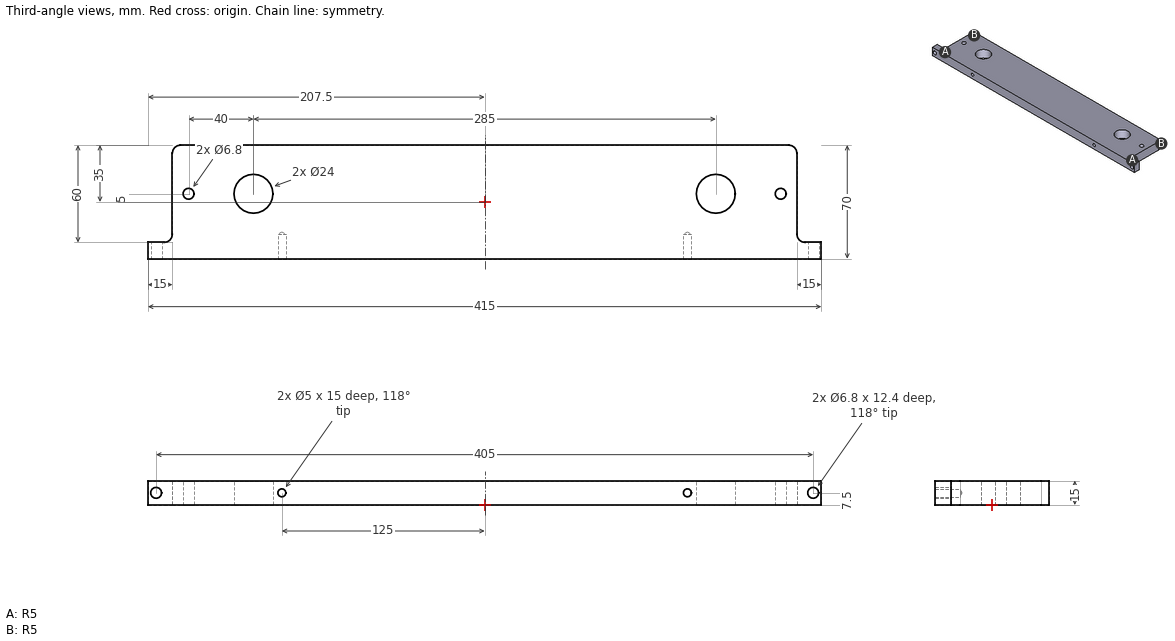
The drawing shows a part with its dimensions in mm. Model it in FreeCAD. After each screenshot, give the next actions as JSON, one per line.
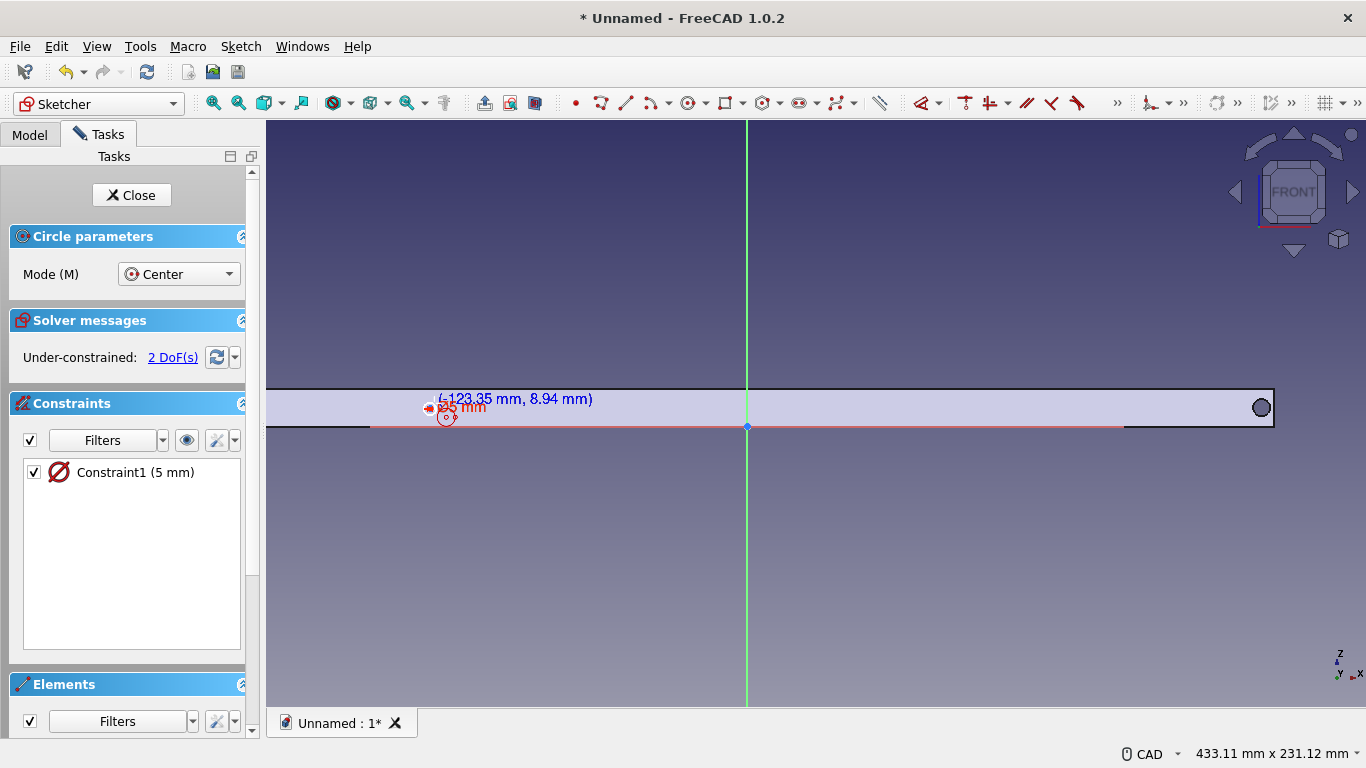
{"action": "scroll", "coordinate": [1065, 408], "scroll_direction": "up", "scroll_amount": 7}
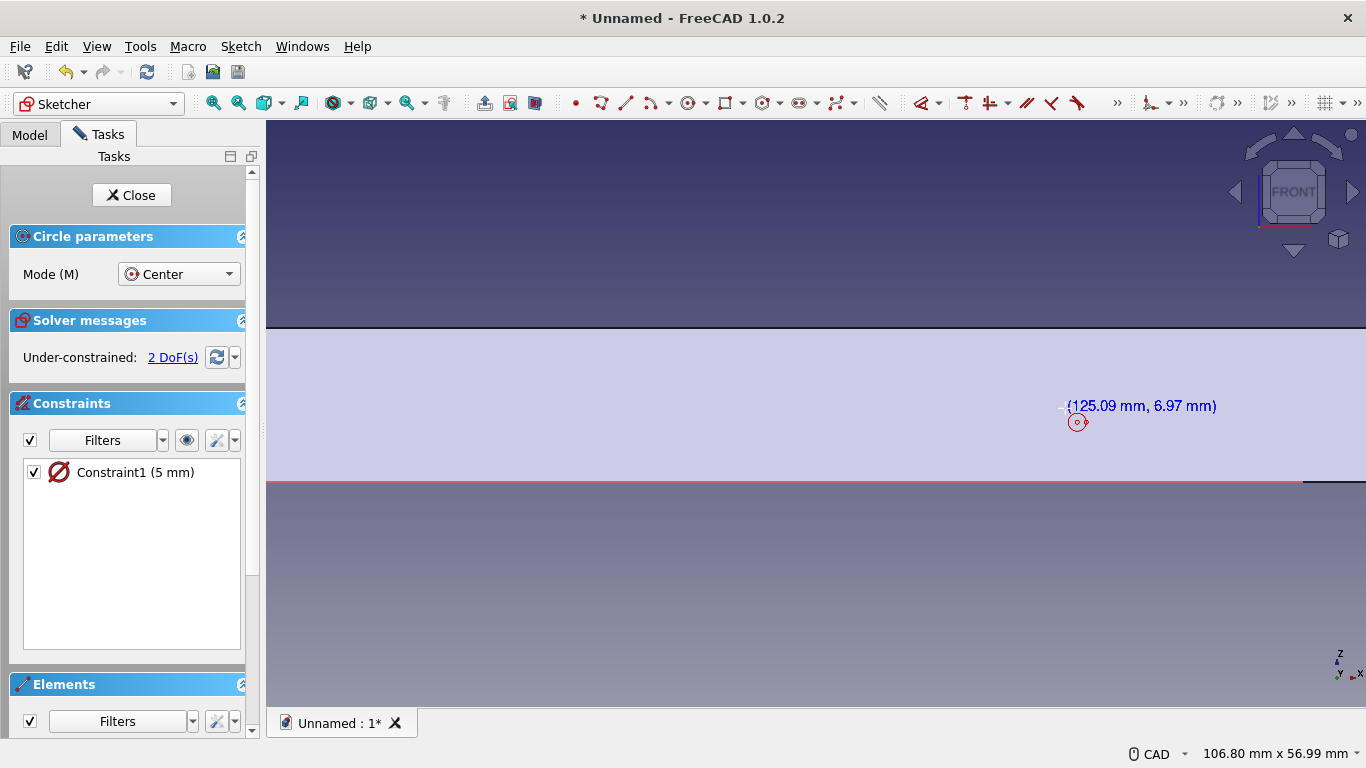
{"action": "scroll", "coordinate": [1066, 408], "scroll_direction": "down", "scroll_amount": 7}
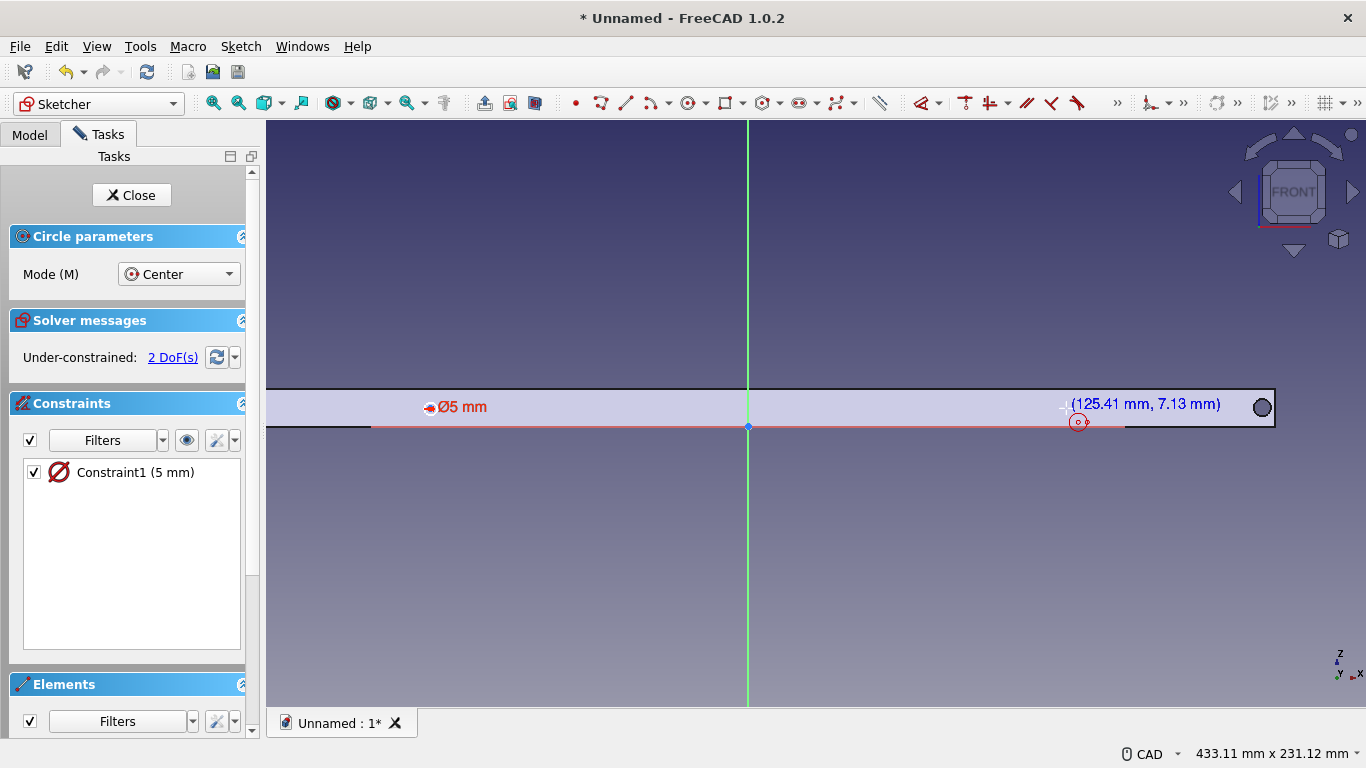
{"action": "left_click", "coordinate": [1066, 408]}
{"action": "mouse_move", "coordinate": [1070, 403]}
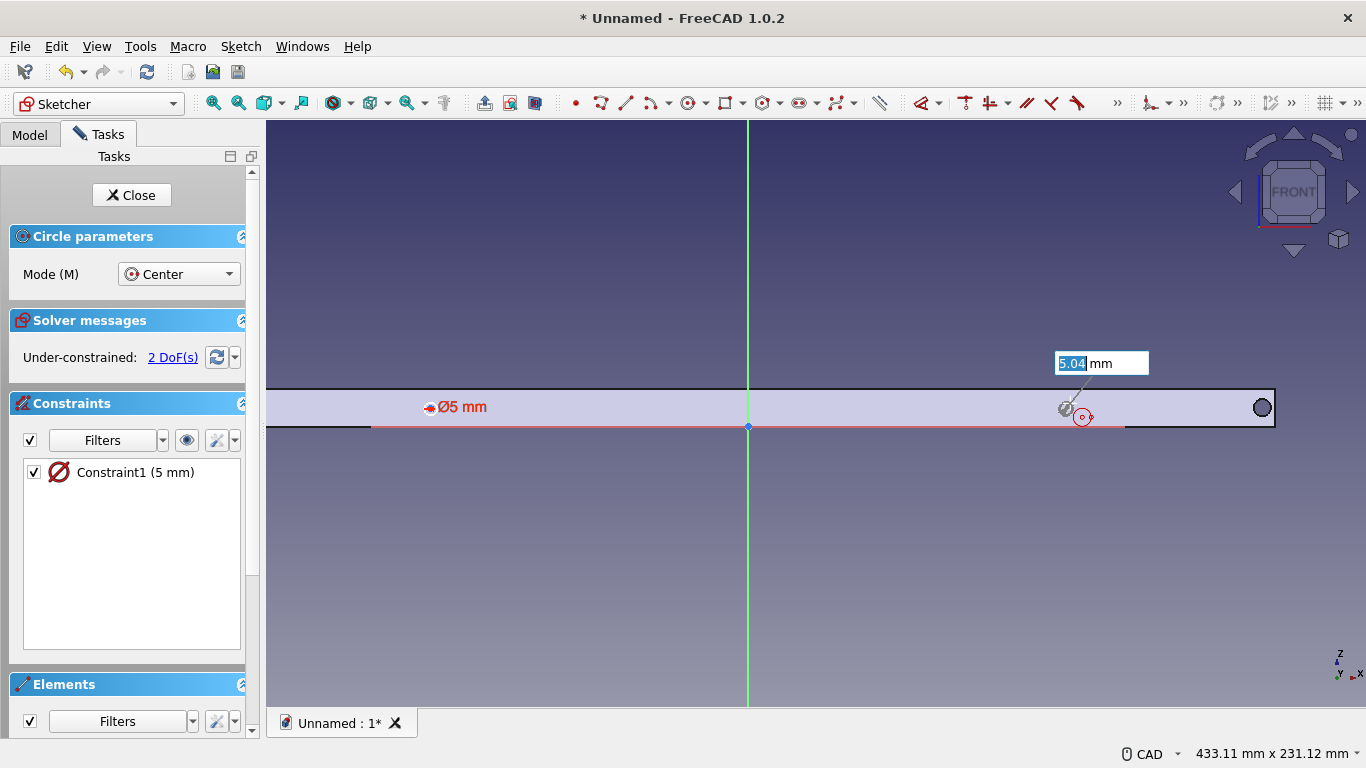
{"action": "type", "text": "5"}
{"action": "key", "text": "Return"}
{"action": "key", "text": "Escape"}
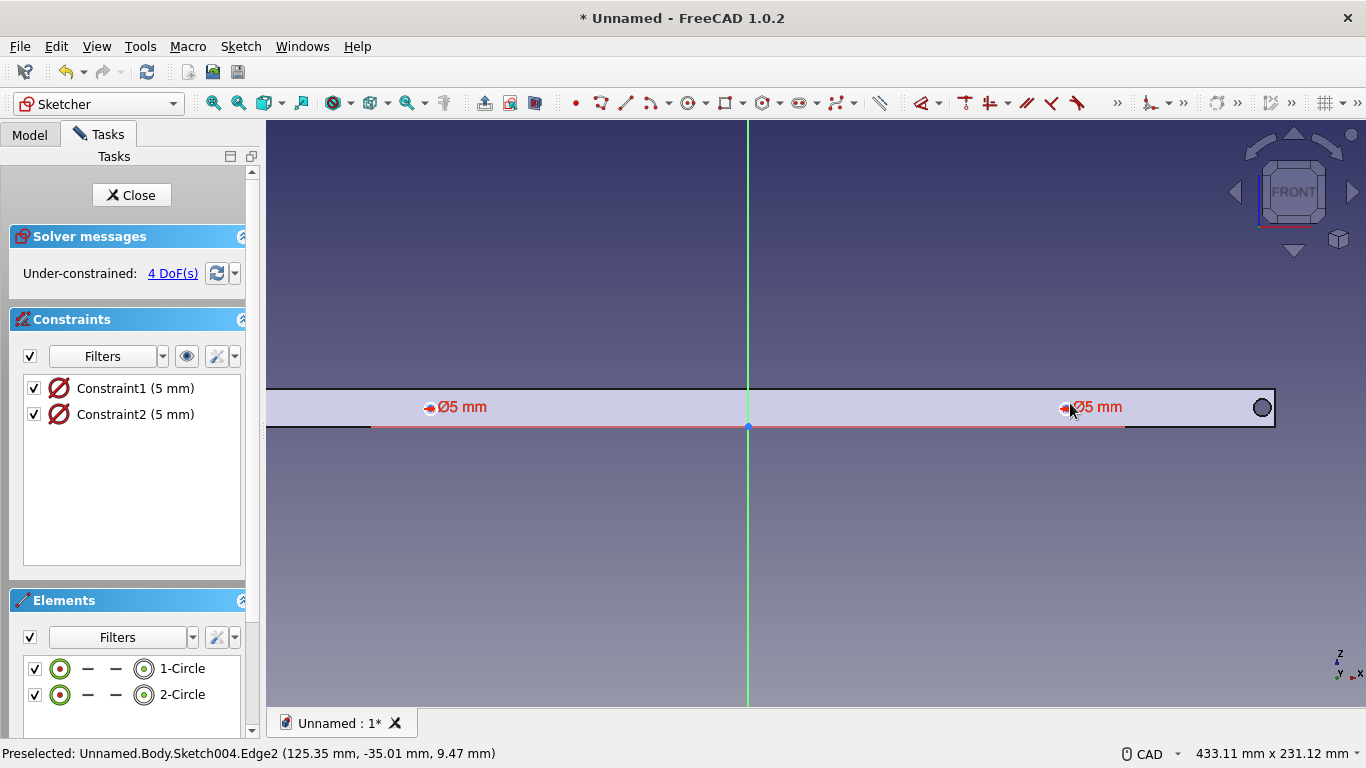
{"action": "left_click", "coordinate": [431, 409]}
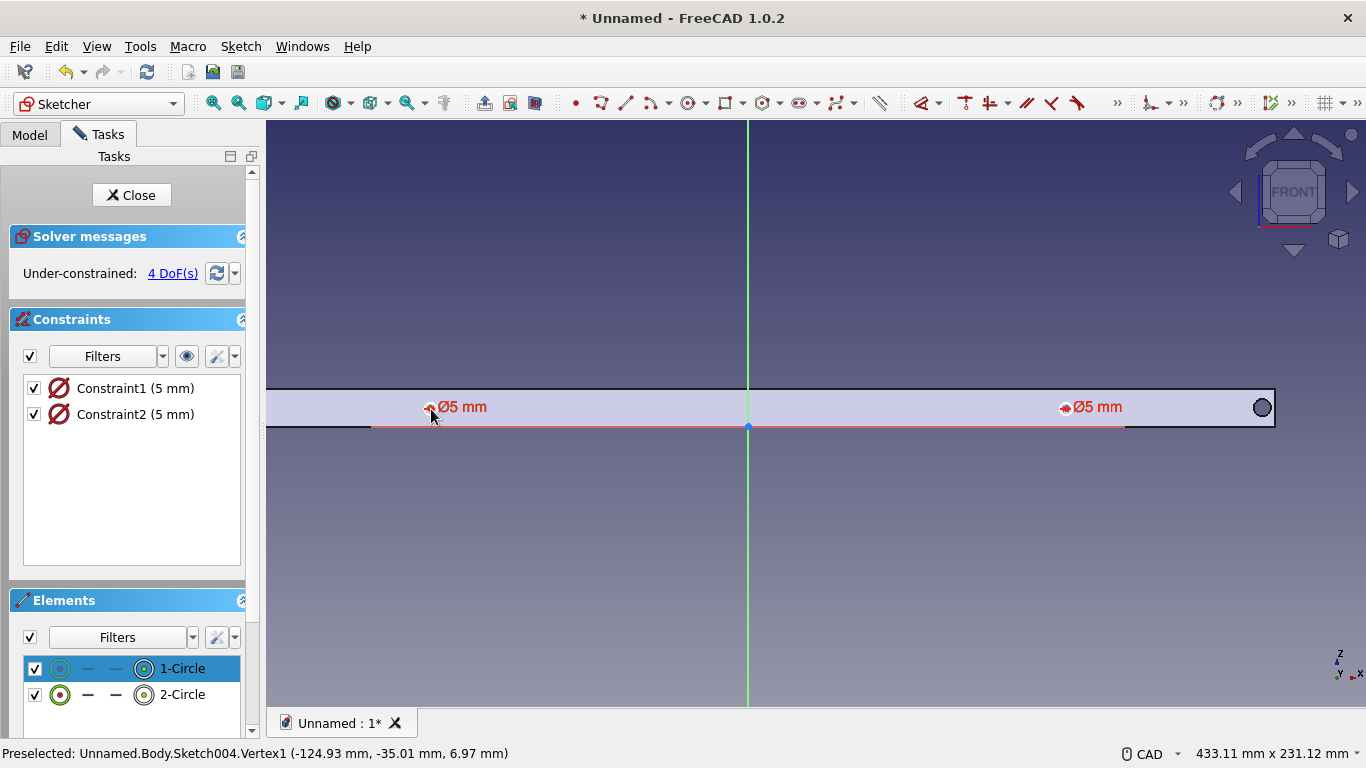
{"action": "left_click", "coordinate": [1066, 409]}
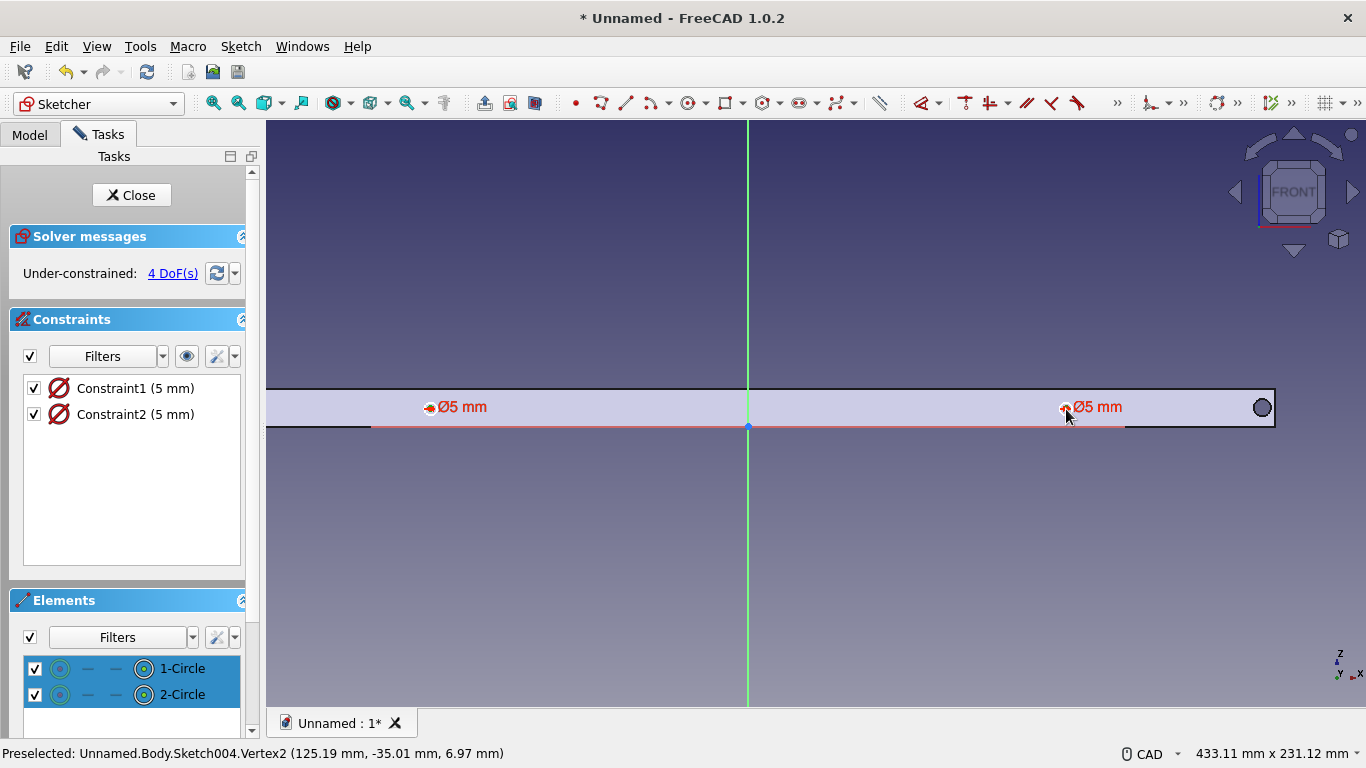
{"action": "left_click", "coordinate": [748, 641]}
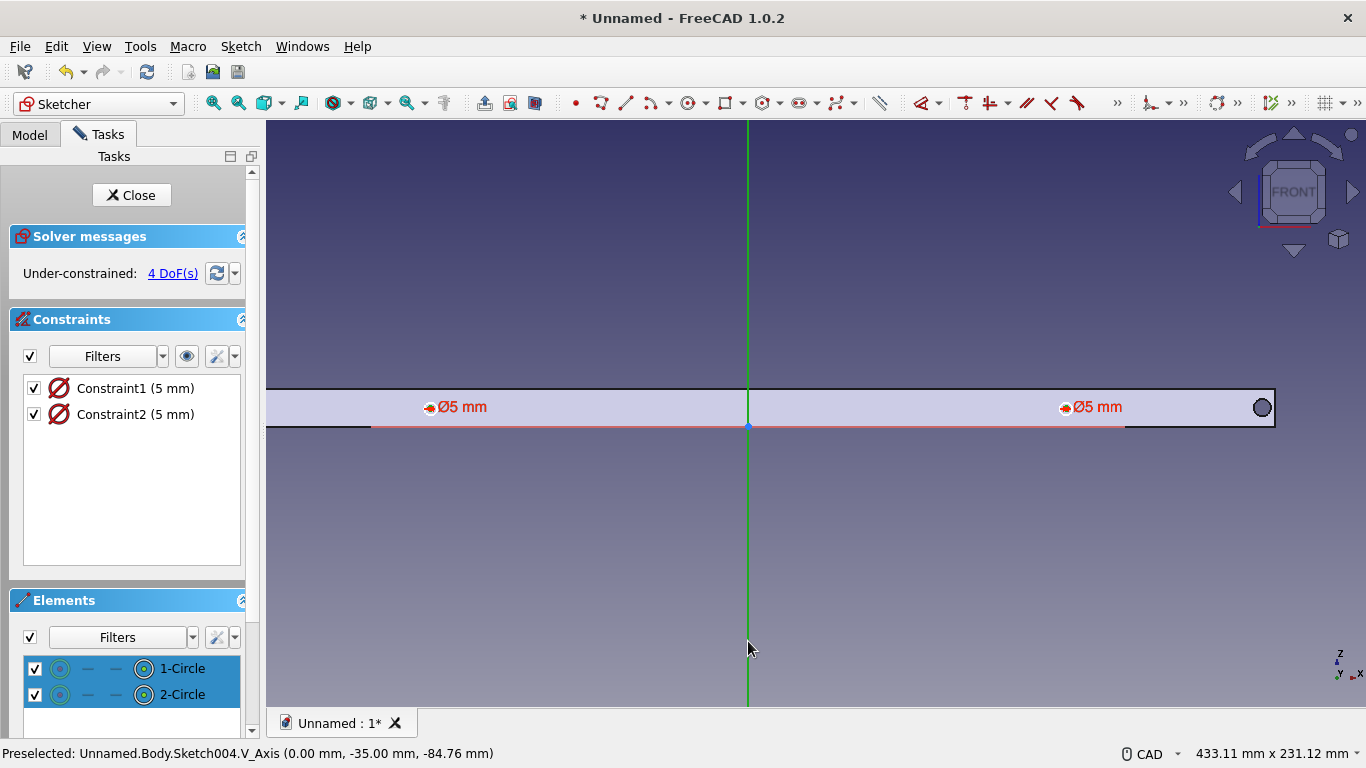
{"action": "key", "text": "s"}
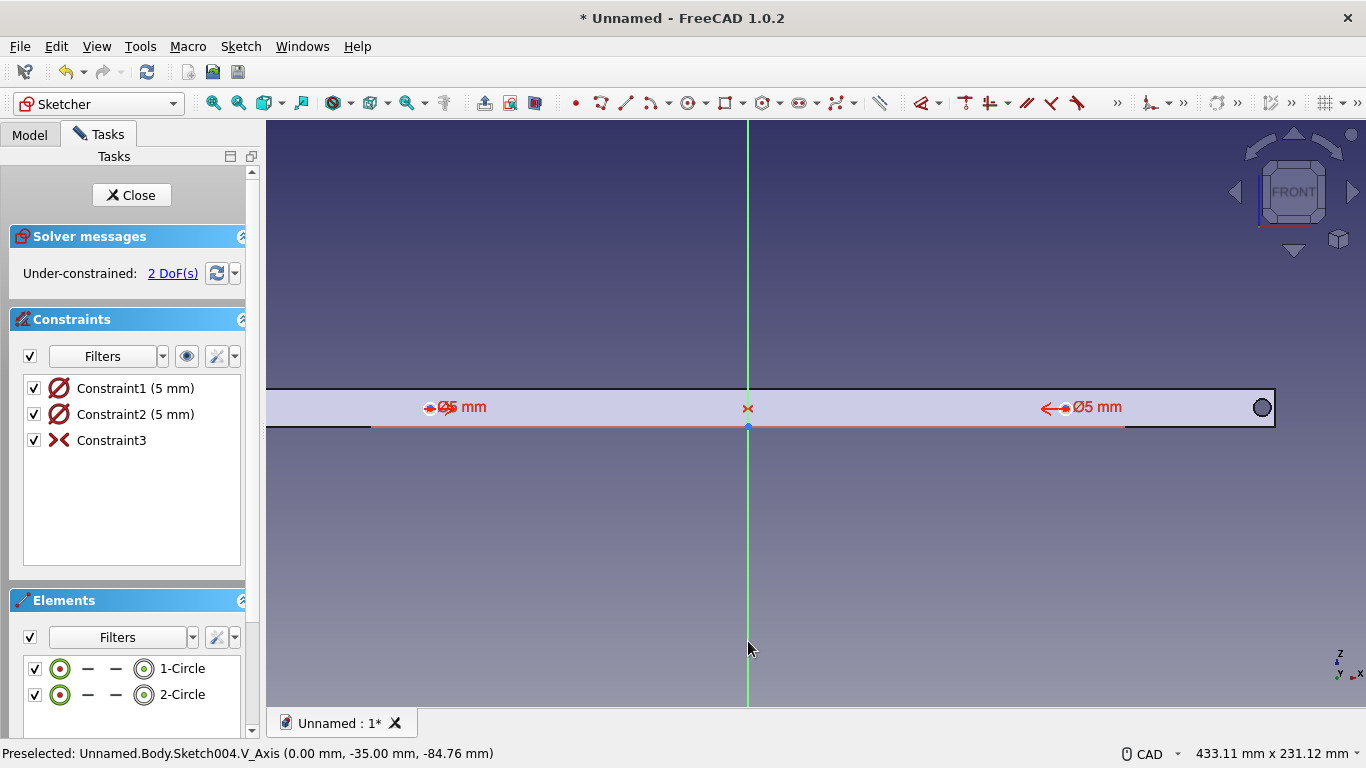
{"action": "key", "text": "d"}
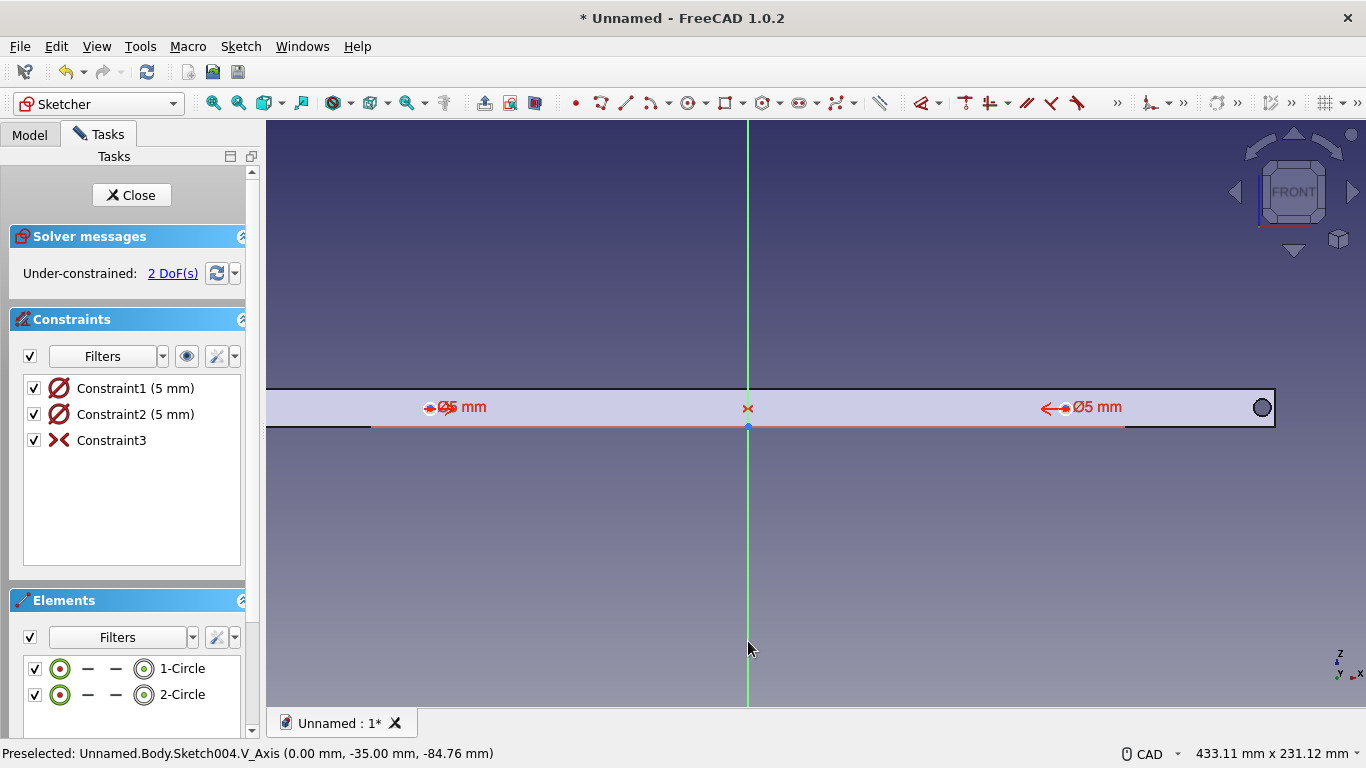
{"action": "left_click", "coordinate": [430, 409]}
{"action": "left_click", "coordinate": [589, 461]}